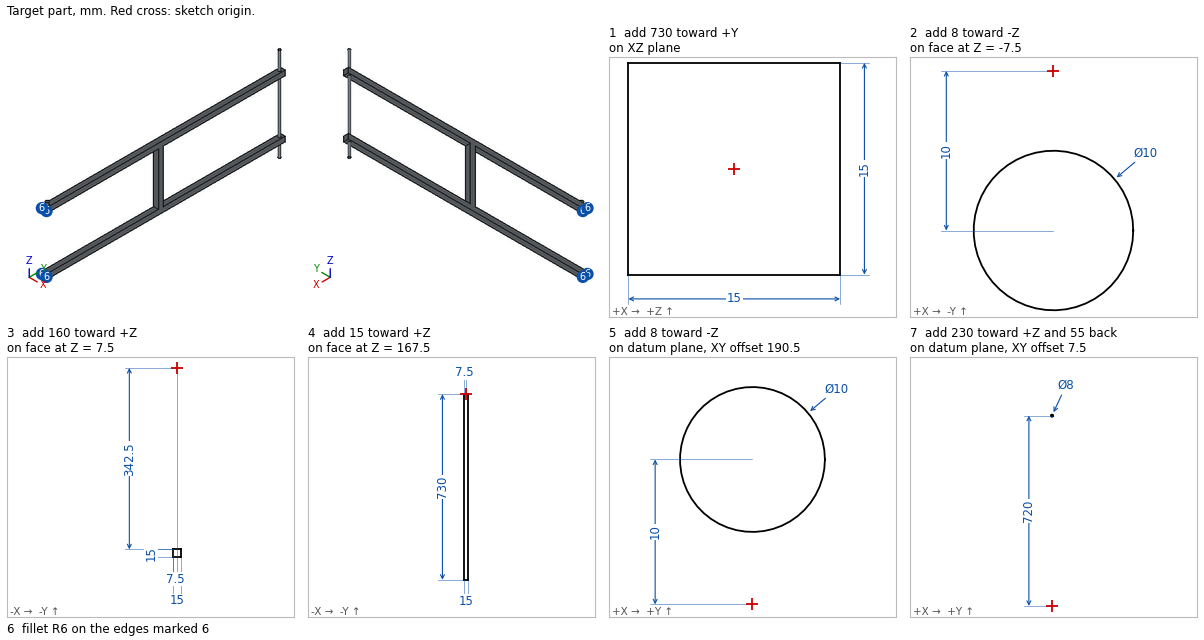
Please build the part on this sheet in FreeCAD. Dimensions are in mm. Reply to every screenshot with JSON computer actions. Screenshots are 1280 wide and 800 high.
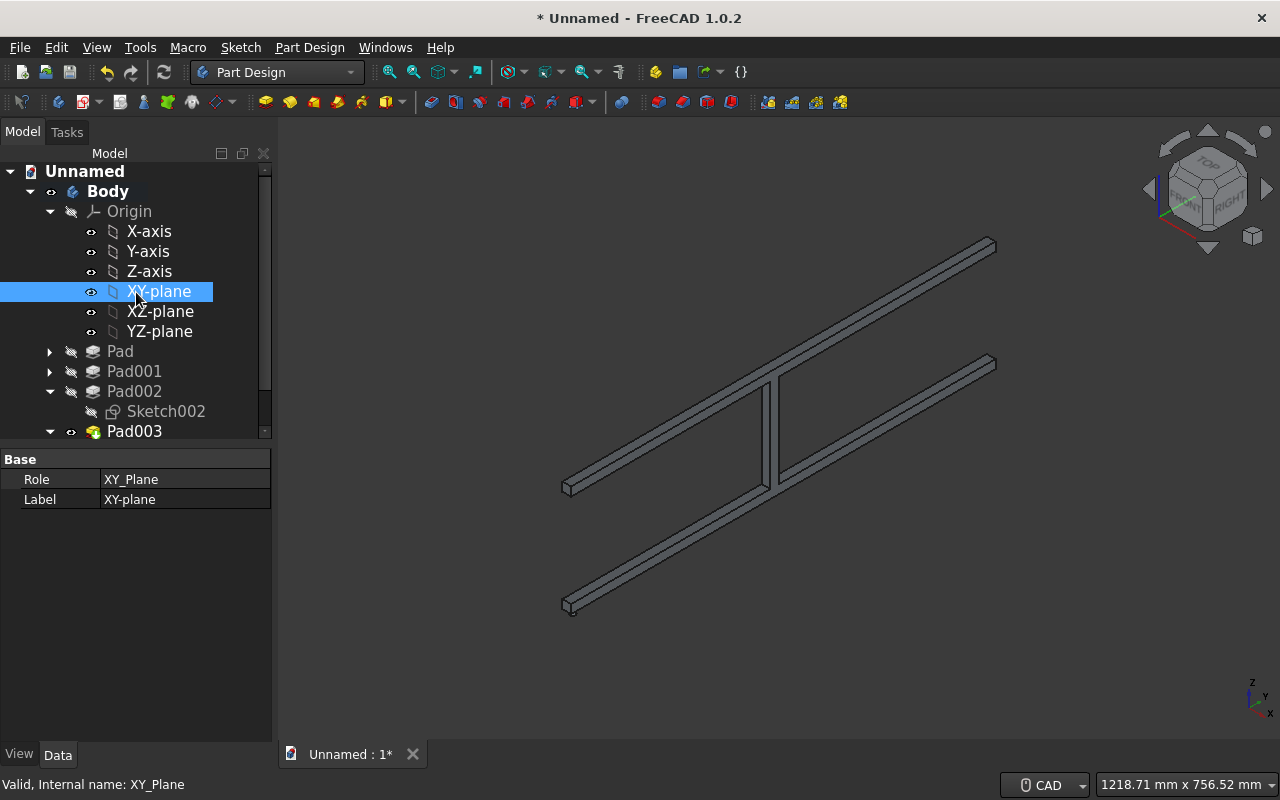
{"action": "left_click", "coordinate": [216, 102]}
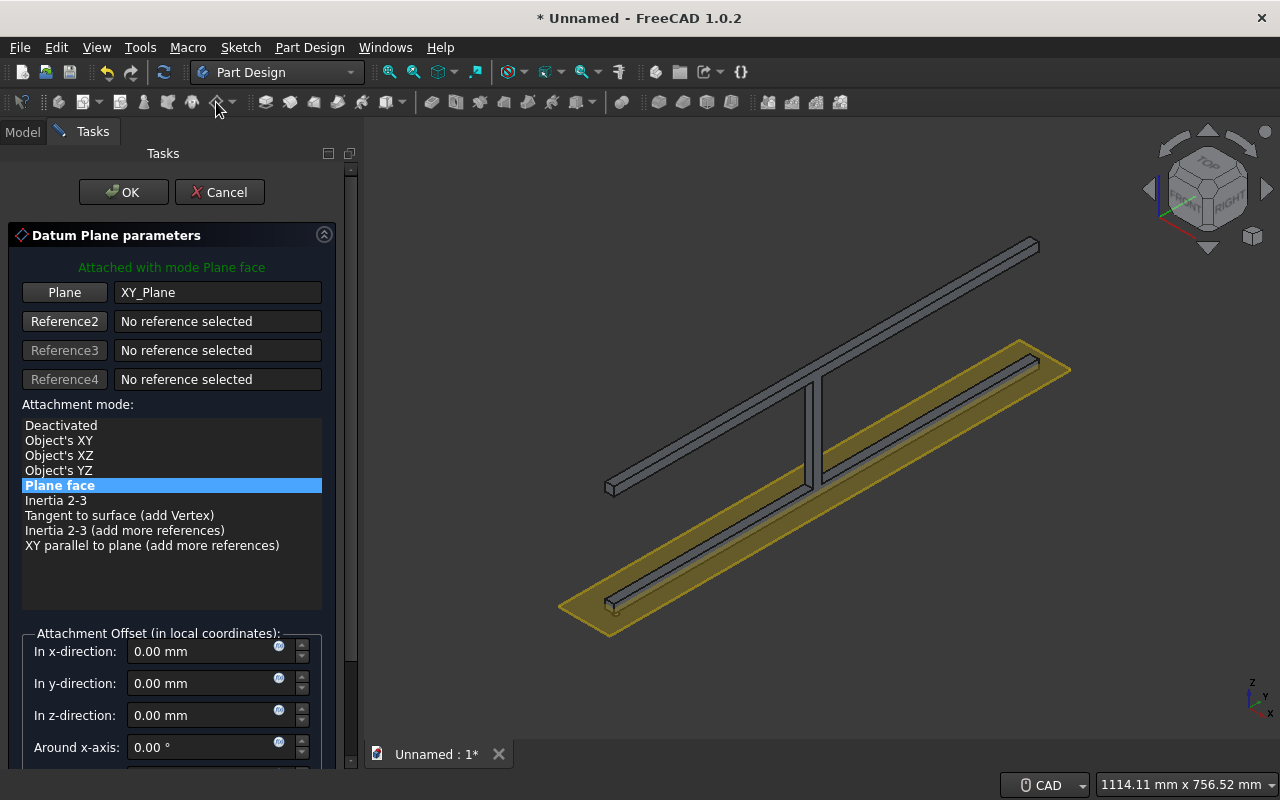
{"action": "triple_click", "coordinate": [210, 715]}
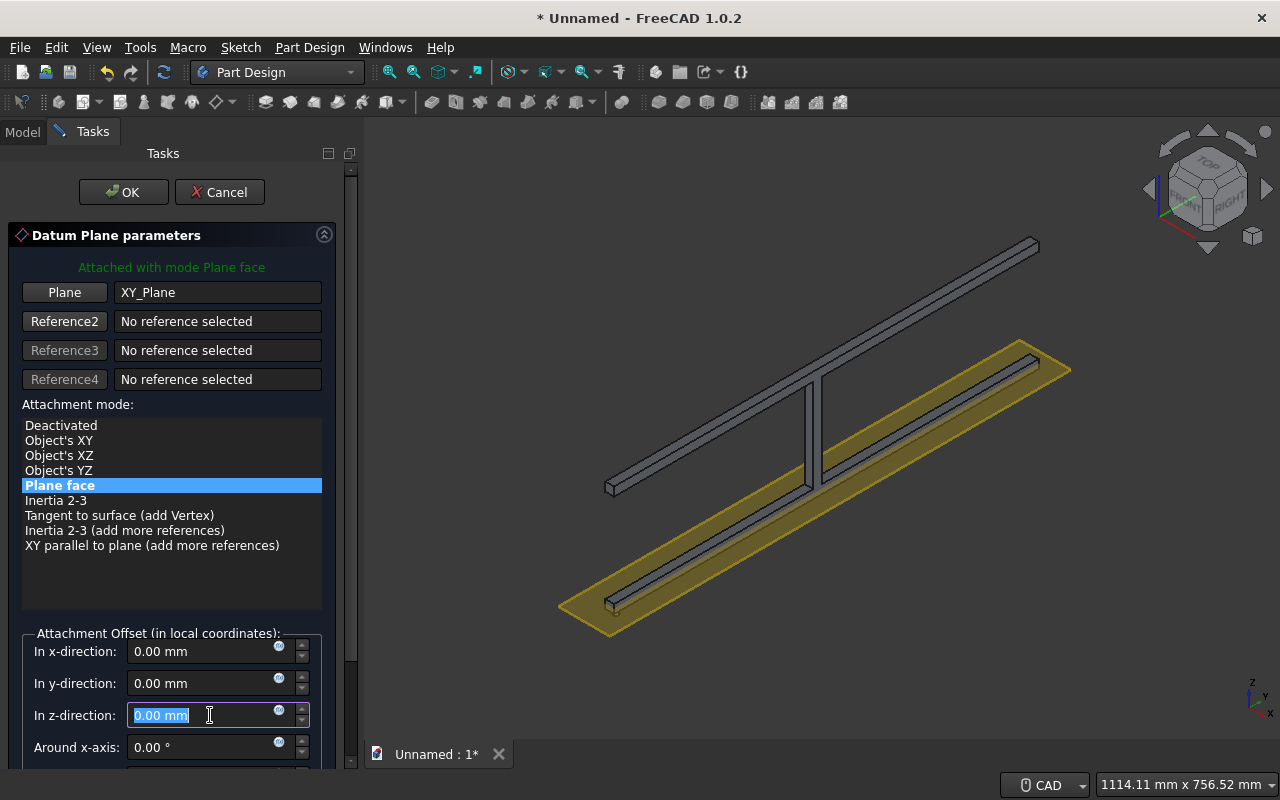
{"action": "type", "text": "190.5"}
{"action": "key", "text": "Tab"}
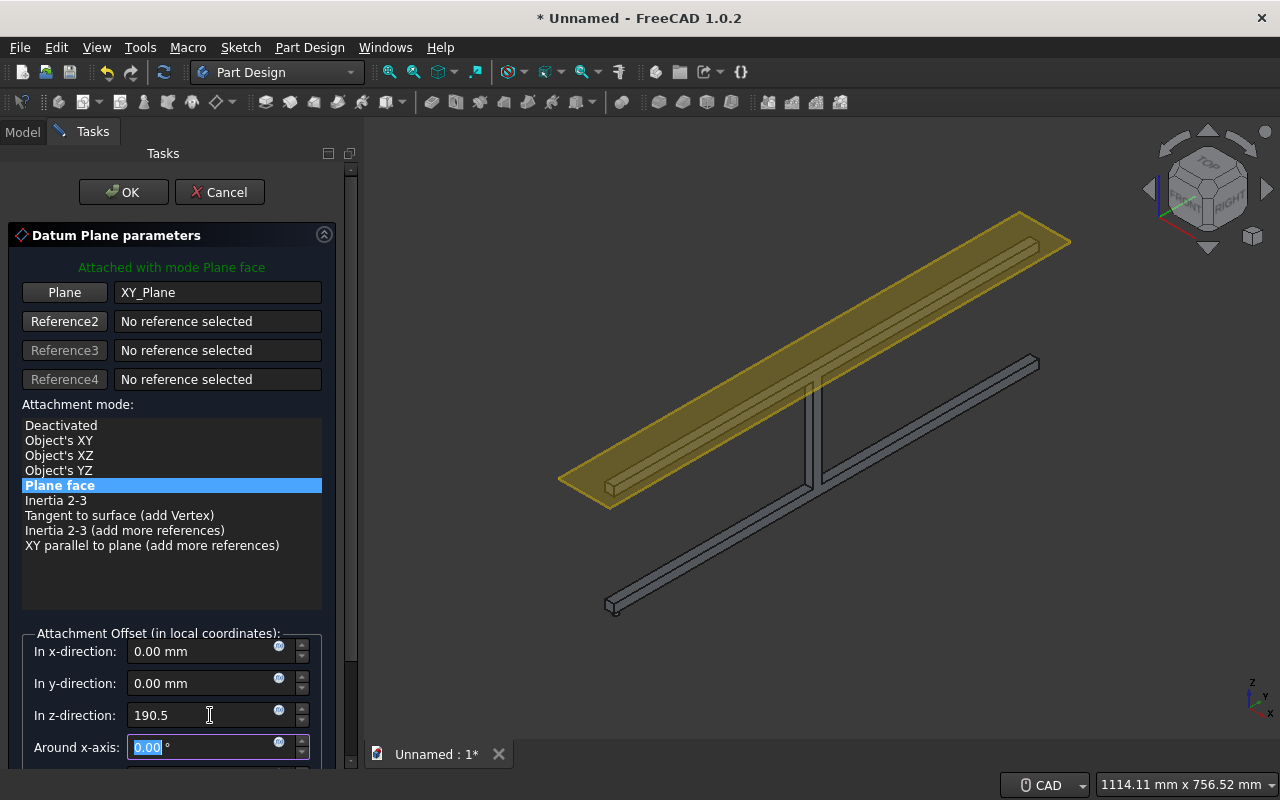
{"action": "left_click", "coordinate": [124, 192]}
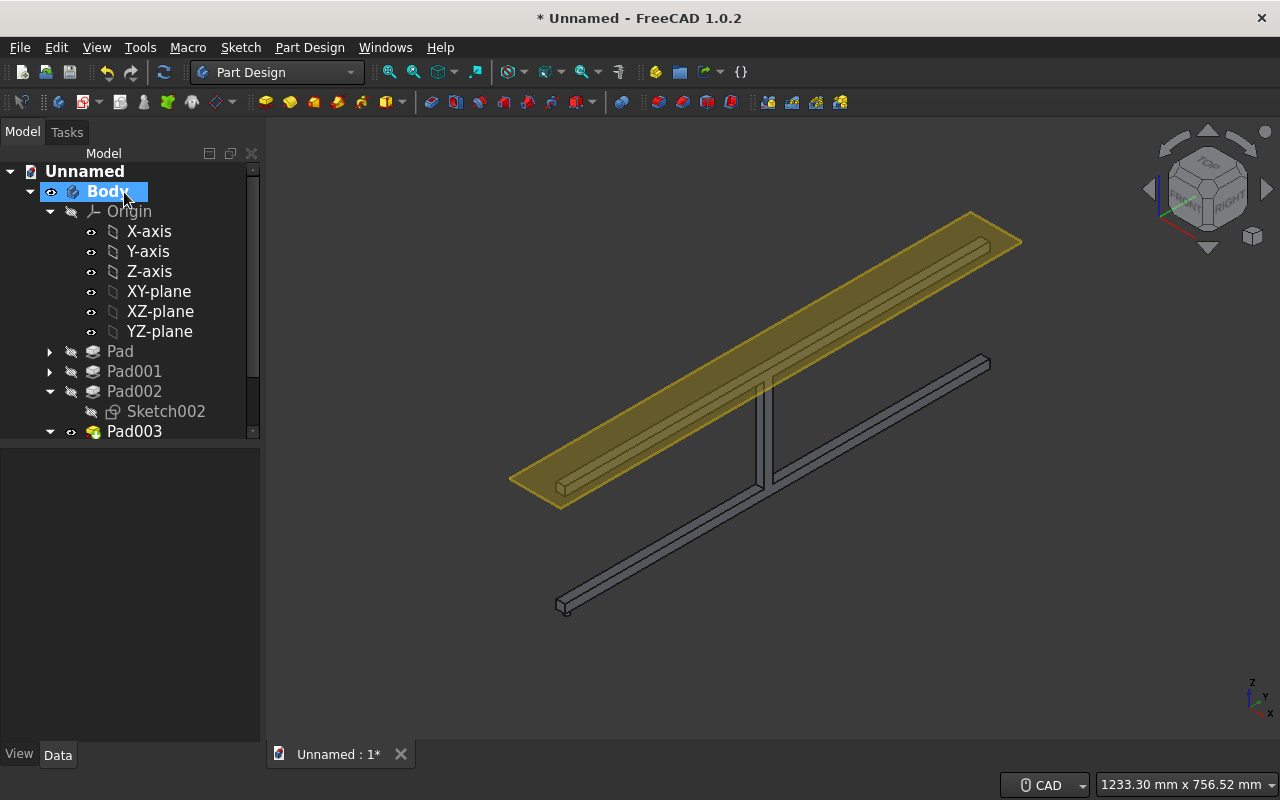
{"action": "scroll", "coordinate": [100, 307], "scroll_direction": "down", "scroll_amount": 3}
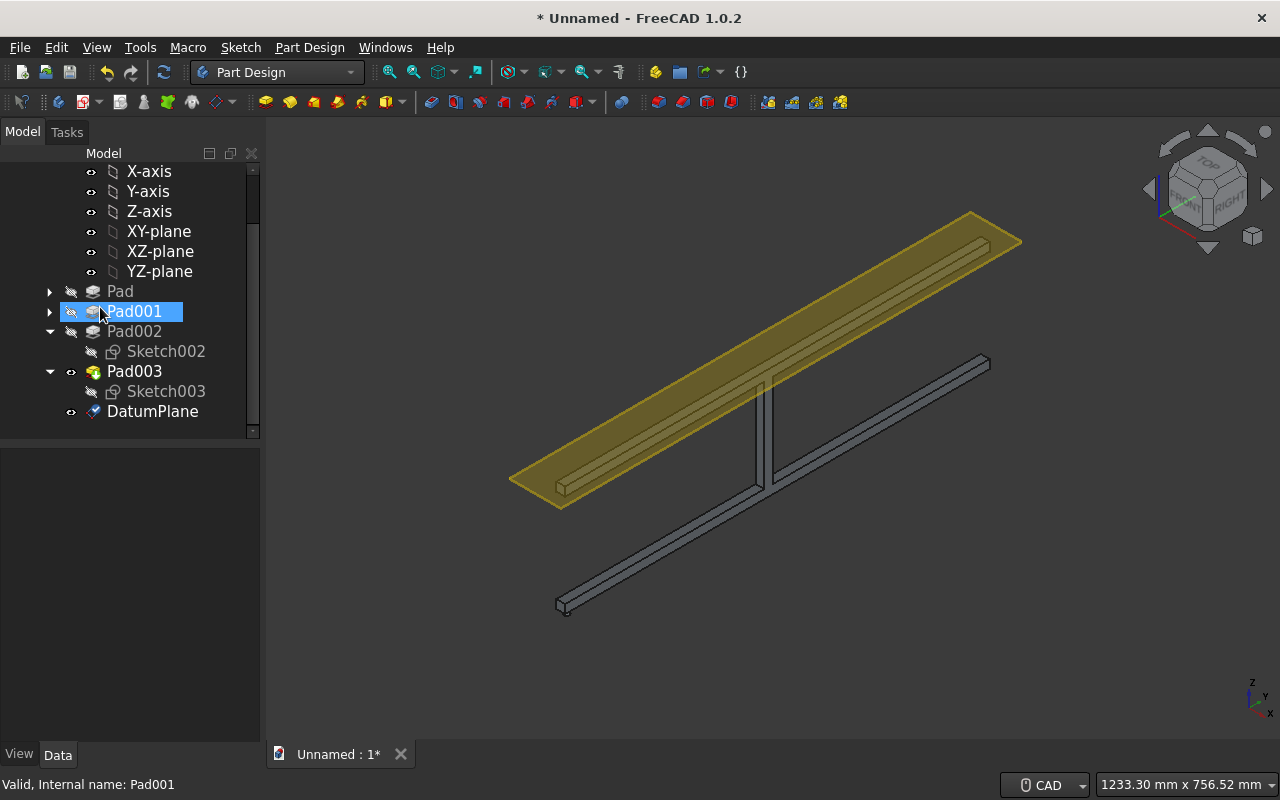
{"action": "left_click", "coordinate": [116, 412]}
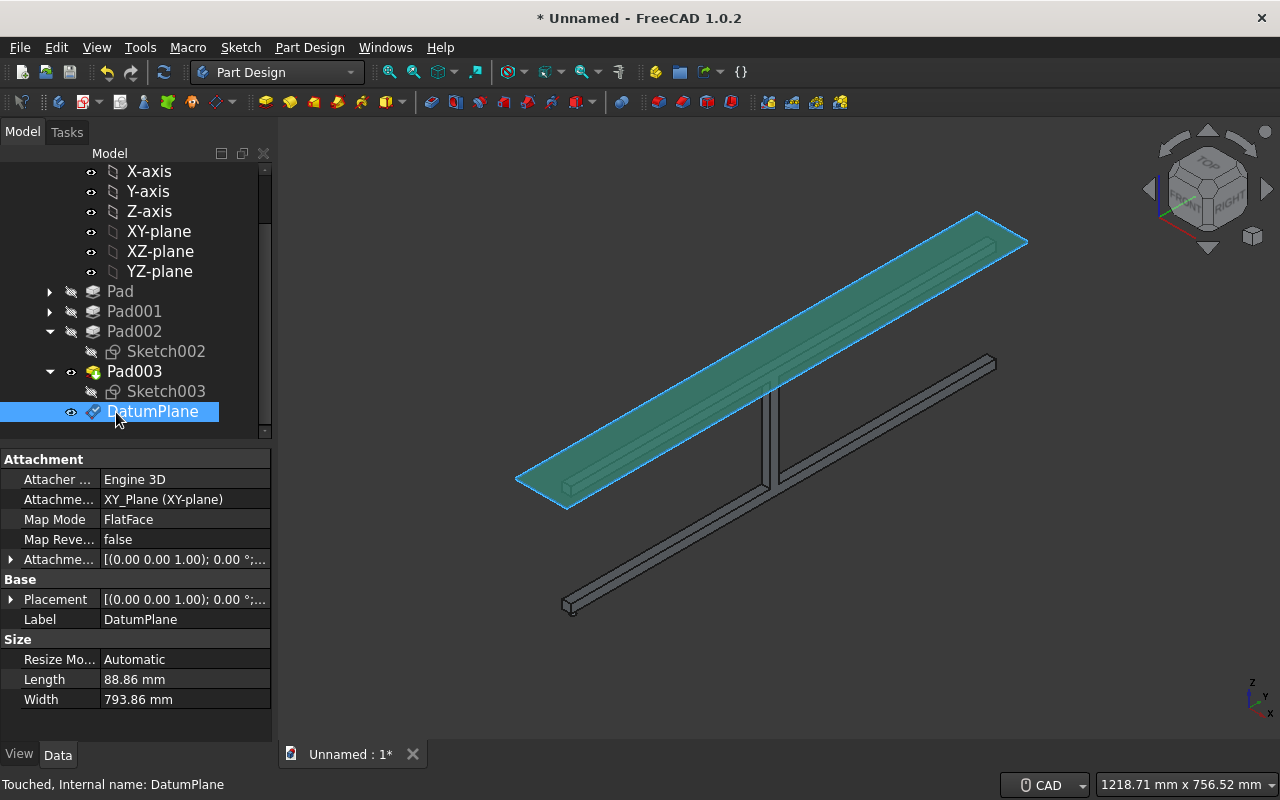
{"action": "left_click", "coordinate": [84, 102]}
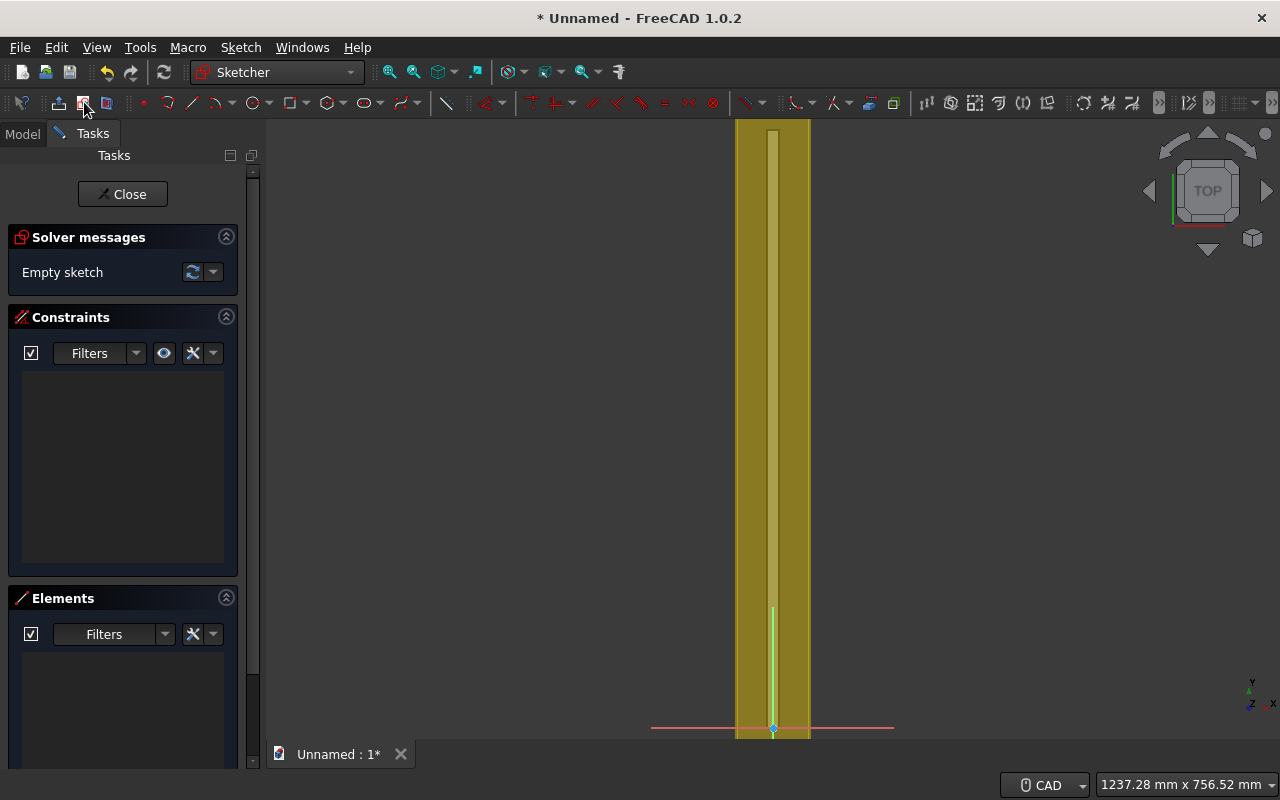
{"action": "scroll", "coordinate": [704, 429], "scroll_direction": "down", "scroll_amount": 5}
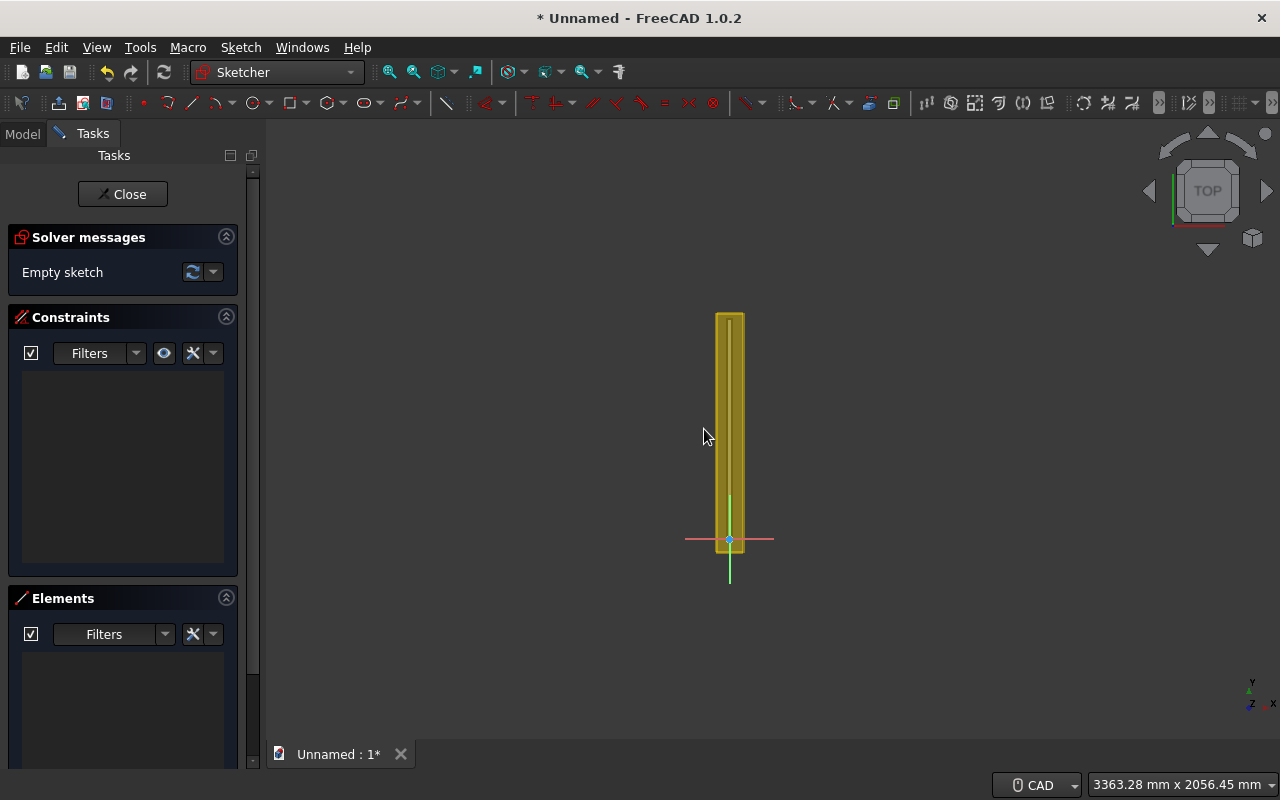
{"action": "scroll", "coordinate": [731, 543], "scroll_direction": "up", "scroll_amount": 15}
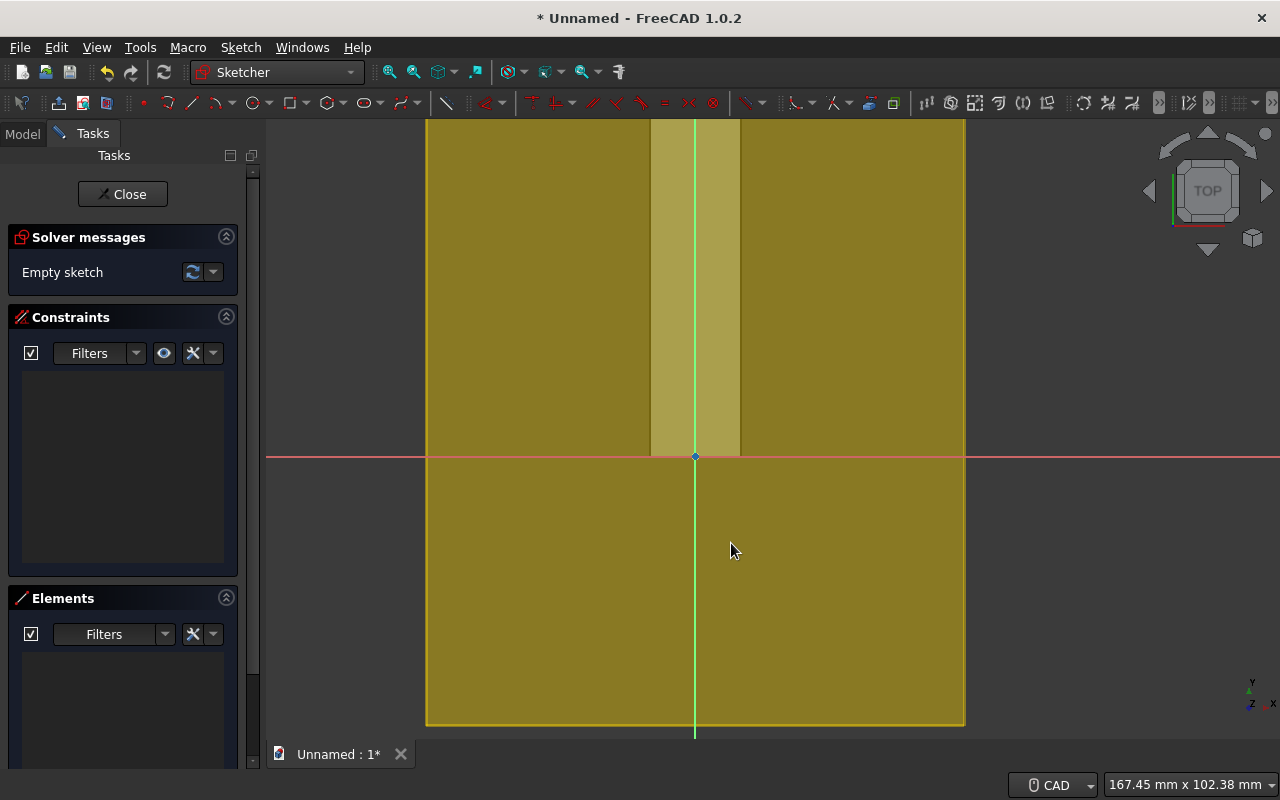
{"action": "scroll", "coordinate": [692, 406], "scroll_direction": "up", "scroll_amount": 7}